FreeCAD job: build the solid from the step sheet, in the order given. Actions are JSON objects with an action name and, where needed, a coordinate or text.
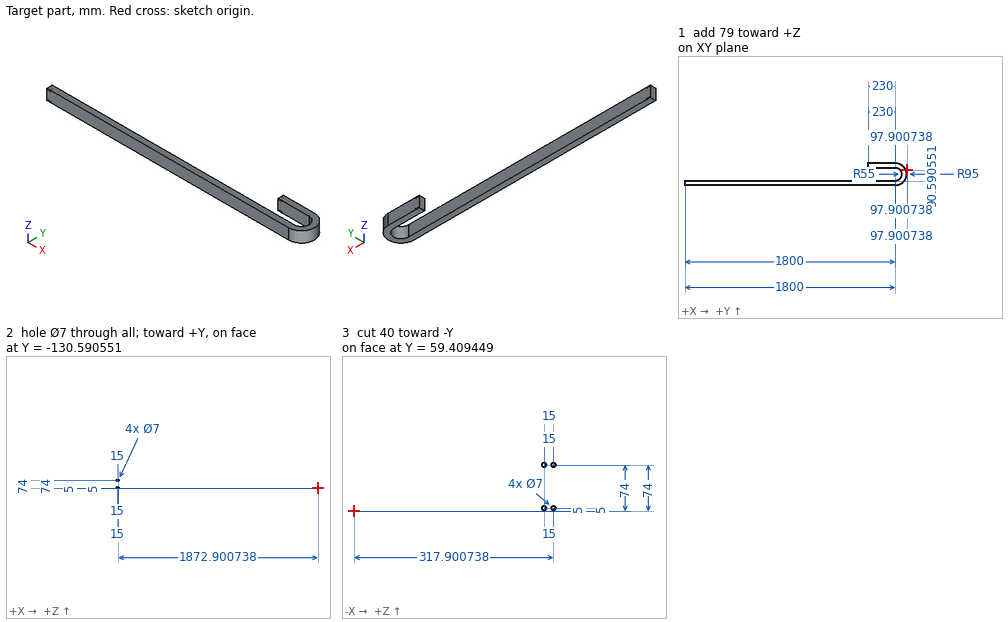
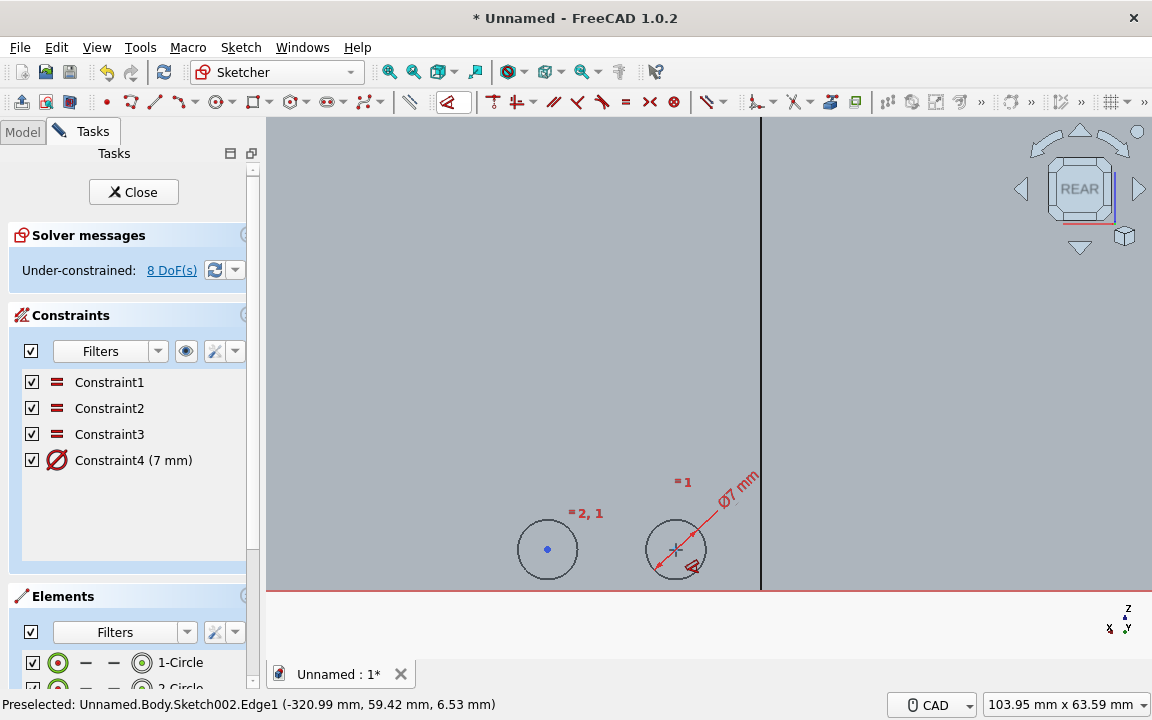
{"action": "left_click", "coordinate": [676, 550]}
{"action": "left_click", "coordinate": [734, 570]}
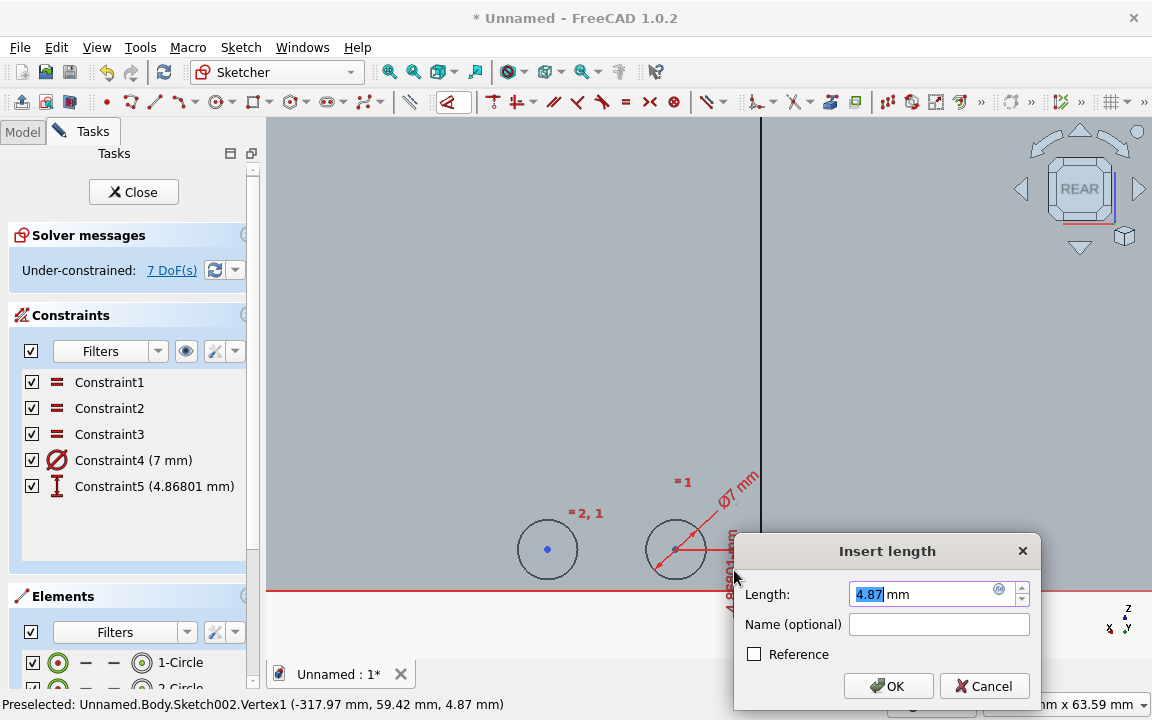
{"action": "type", "text": "5"}
{"action": "key", "text": "Return"}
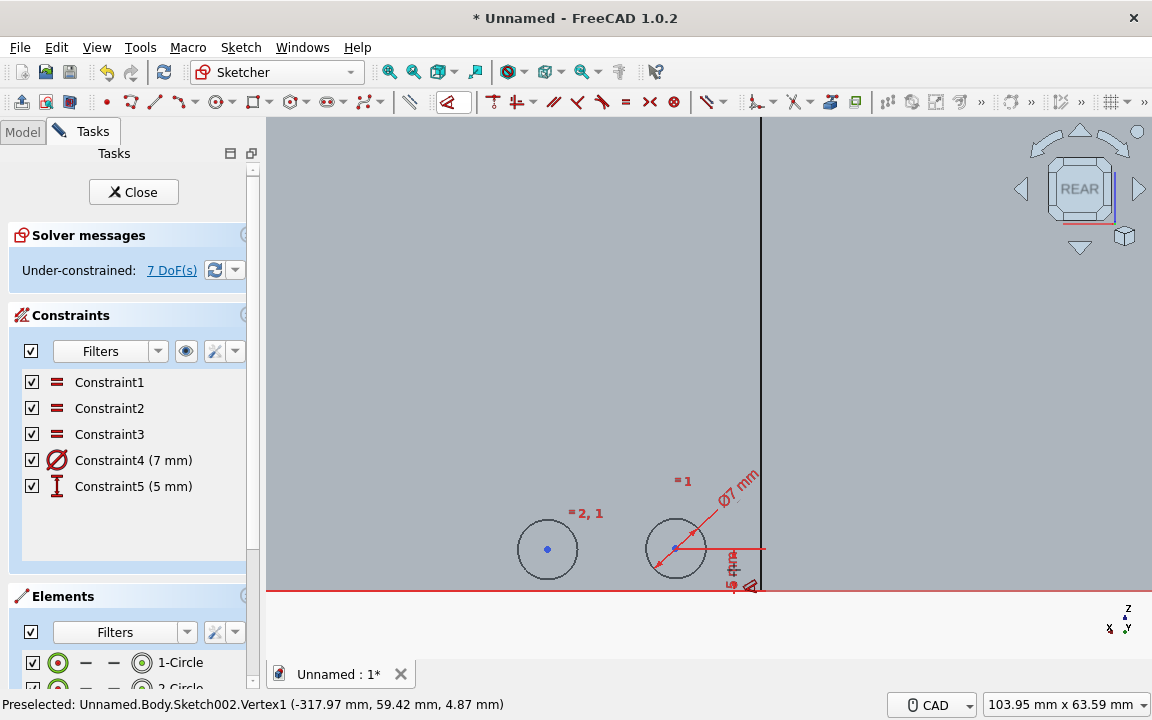
{"action": "left_click", "coordinate": [548, 550]}
{"action": "left_click", "coordinate": [606, 570]}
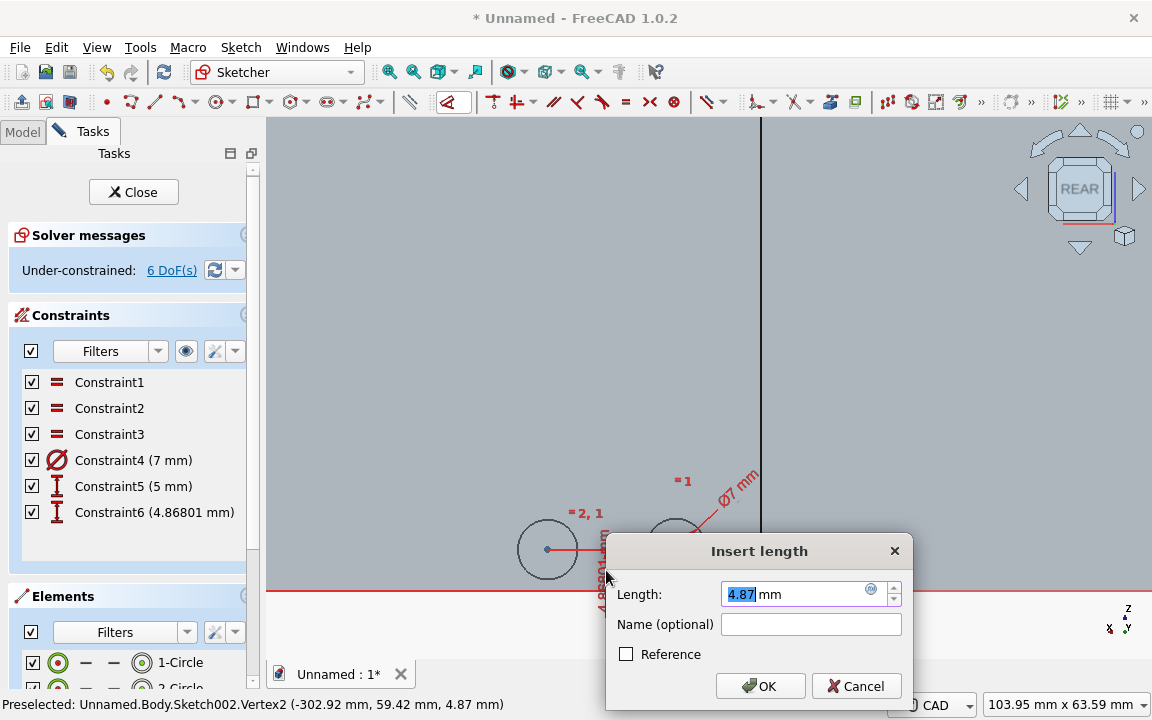
{"action": "type", "text": "5"}
{"action": "key", "text": "Return"}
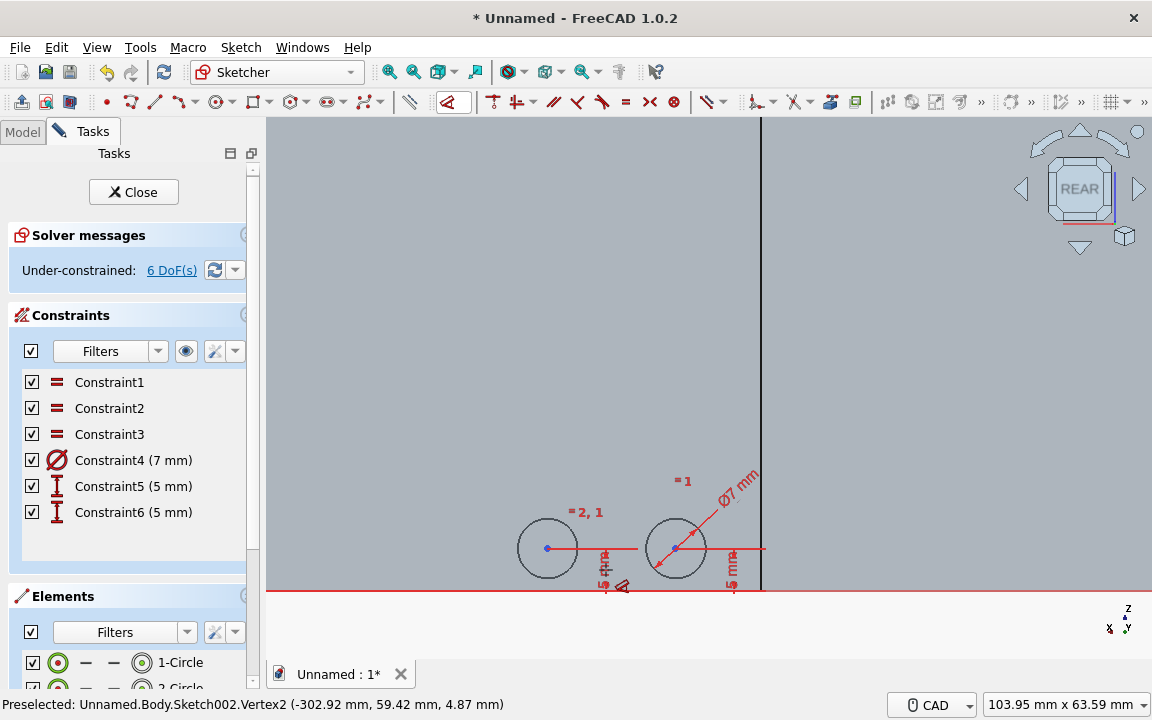
{"action": "scroll", "coordinate": [676, 550], "scroll_direction": "down", "scroll_amount": 3}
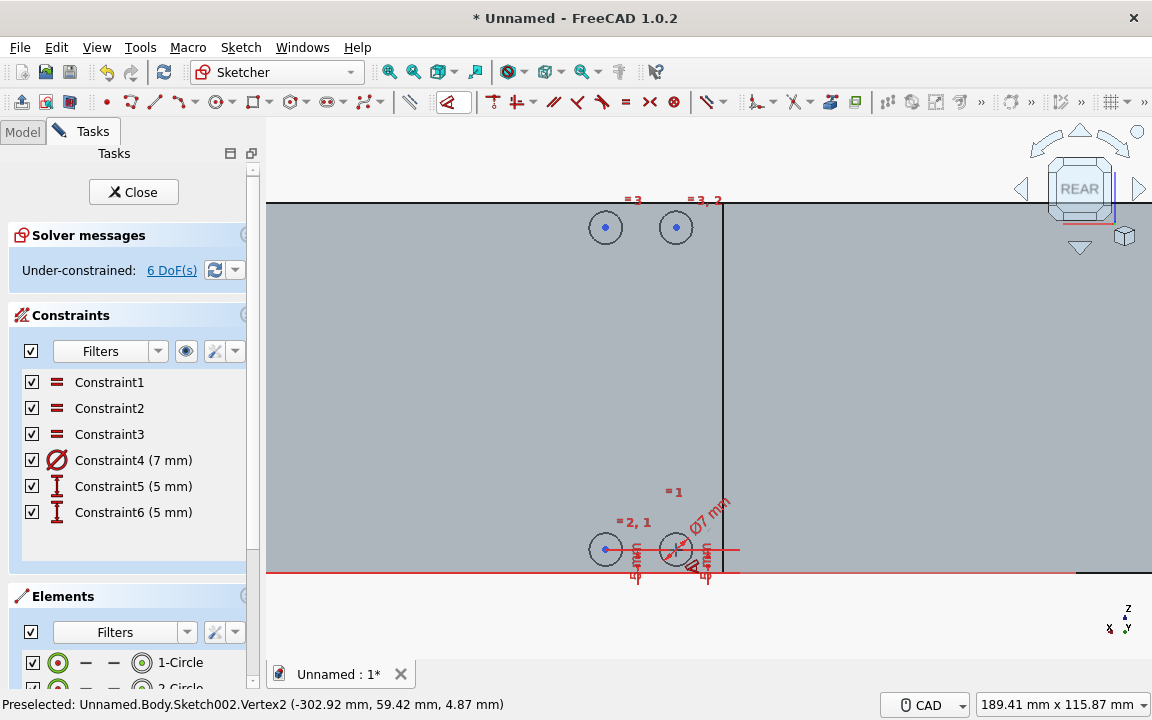
{"action": "left_click", "coordinate": [676, 228]}
{"action": "left_click", "coordinate": [710, 400]}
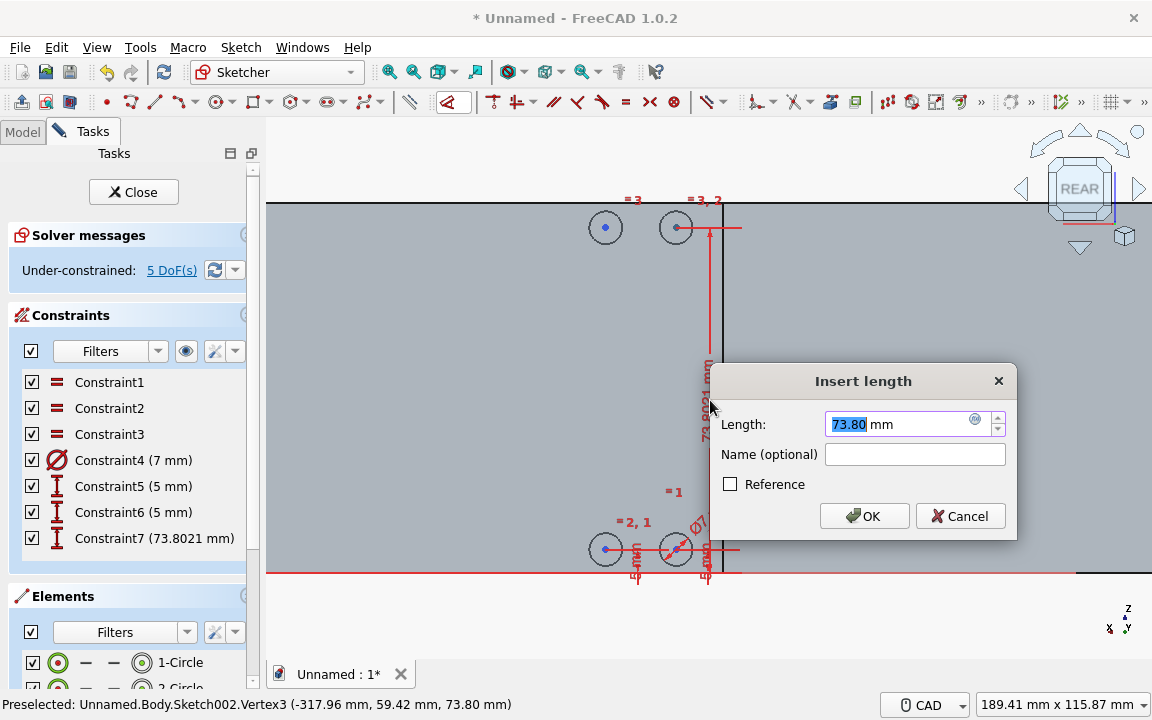
{"action": "type", "text": "74"}
{"action": "key", "text": "Return"}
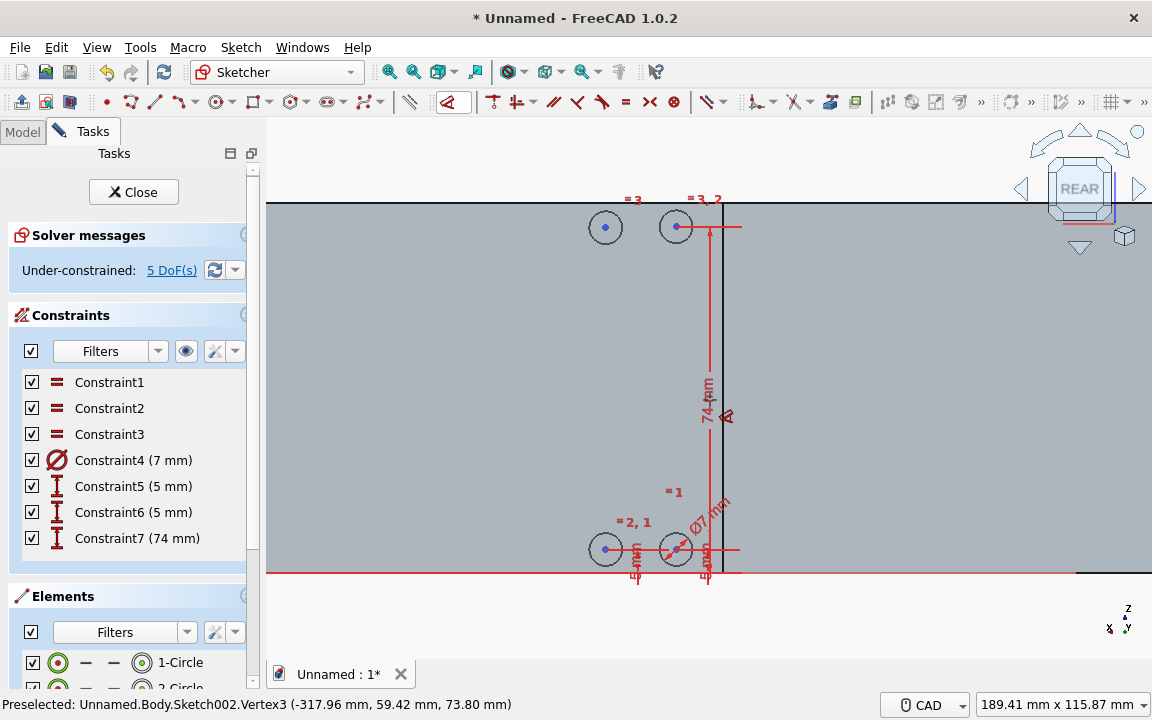
{"action": "left_click", "coordinate": [606, 228]}
{"action": "left_click", "coordinate": [640, 400]}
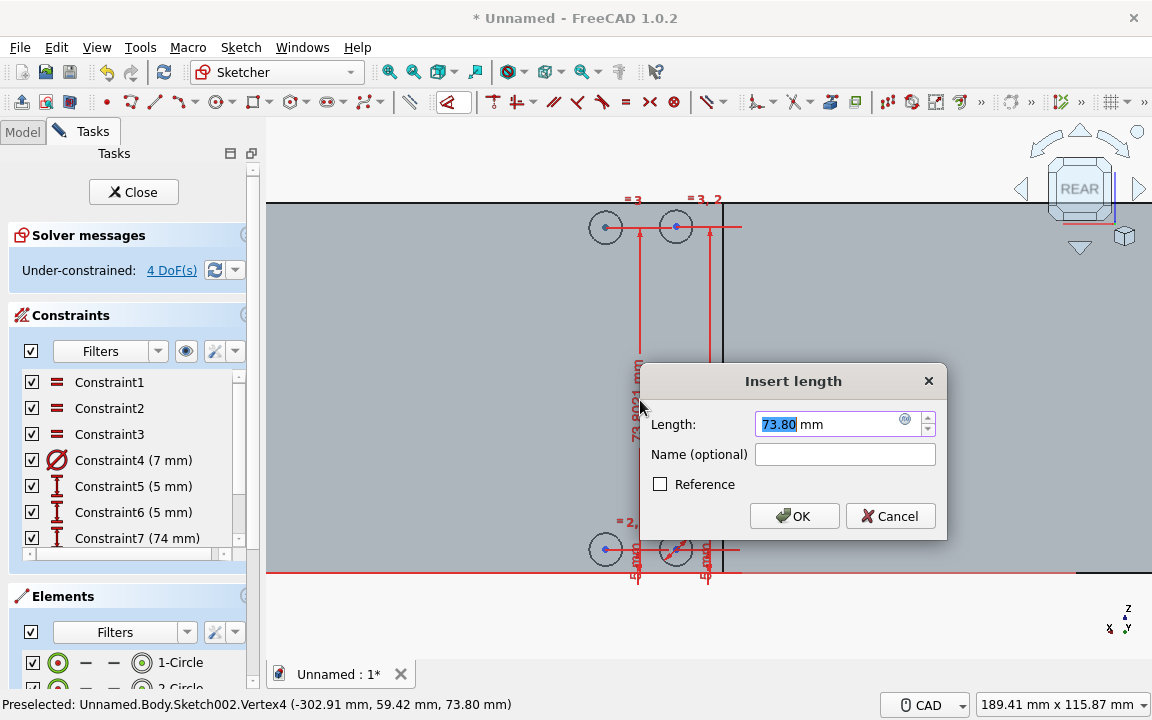
{"action": "type", "text": "74"}
{"action": "key", "text": "Return"}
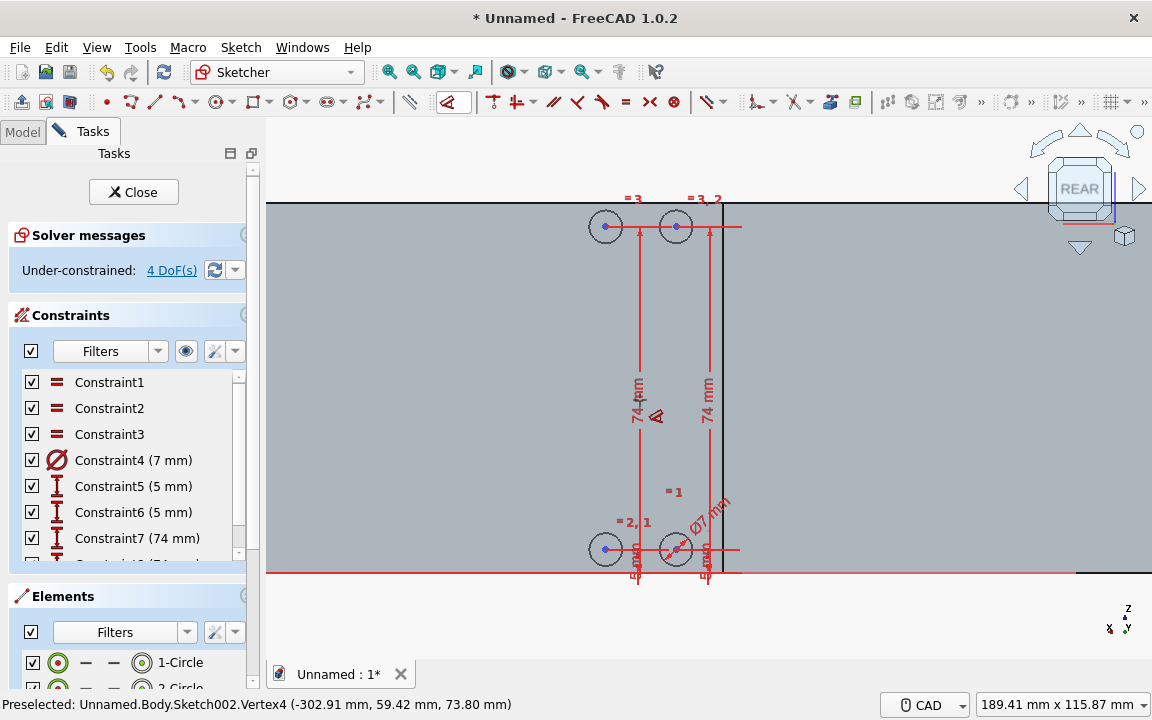
{"action": "left_click", "coordinate": [676, 550]}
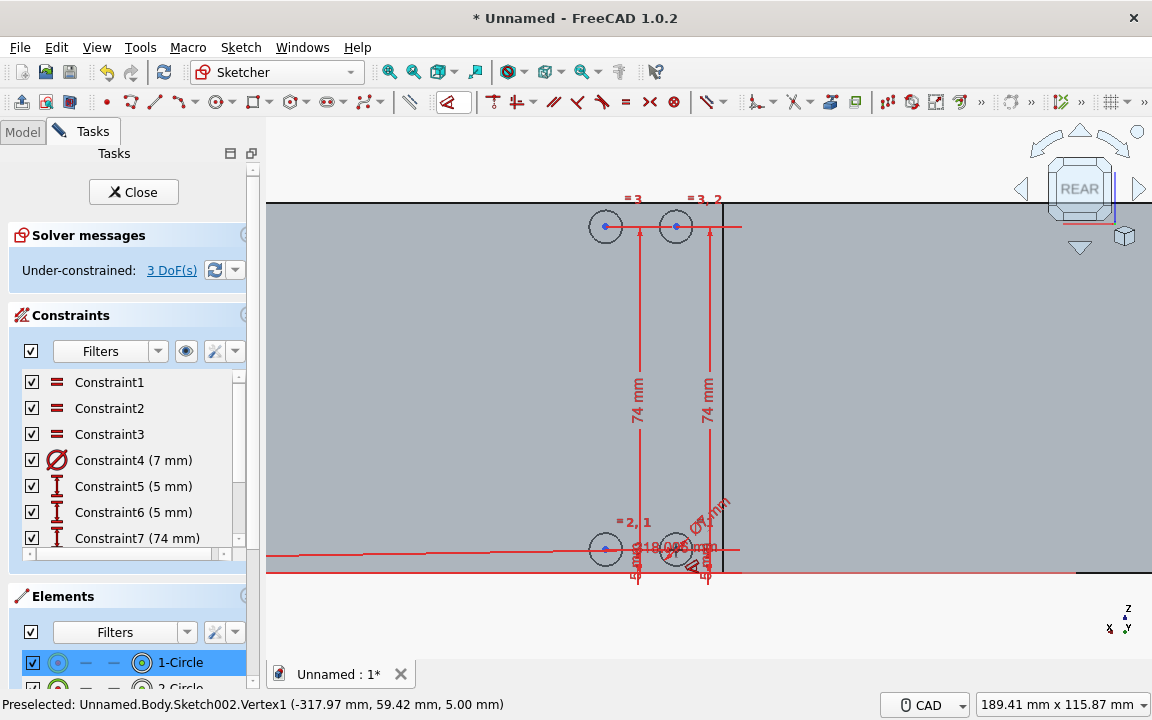
{"action": "left_click", "coordinate": [606, 550]}
{"action": "left_click", "coordinate": [641, 516]}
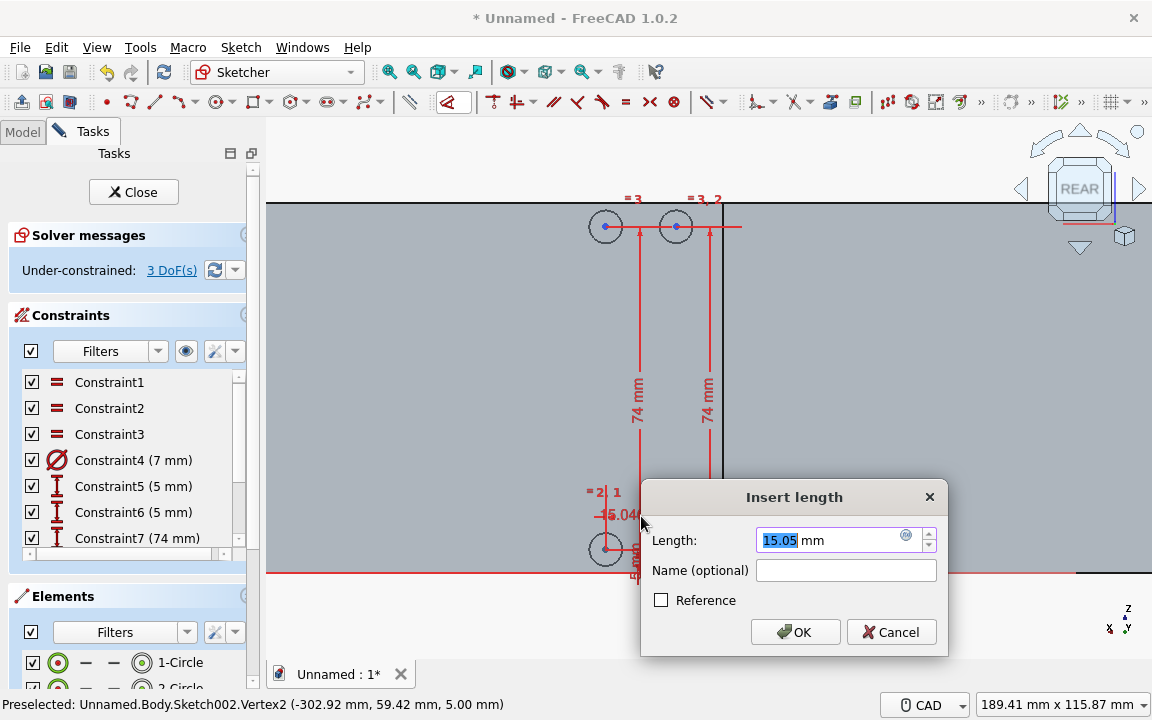
{"action": "type", "text": "15"}
{"action": "key", "text": "Return"}